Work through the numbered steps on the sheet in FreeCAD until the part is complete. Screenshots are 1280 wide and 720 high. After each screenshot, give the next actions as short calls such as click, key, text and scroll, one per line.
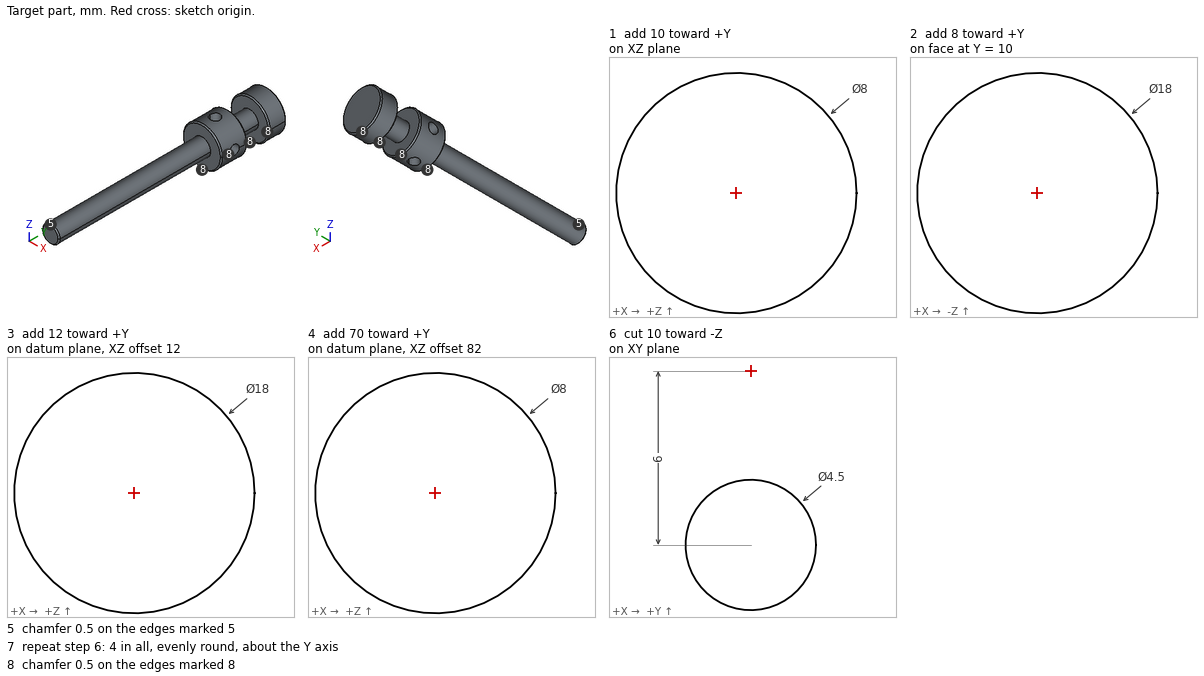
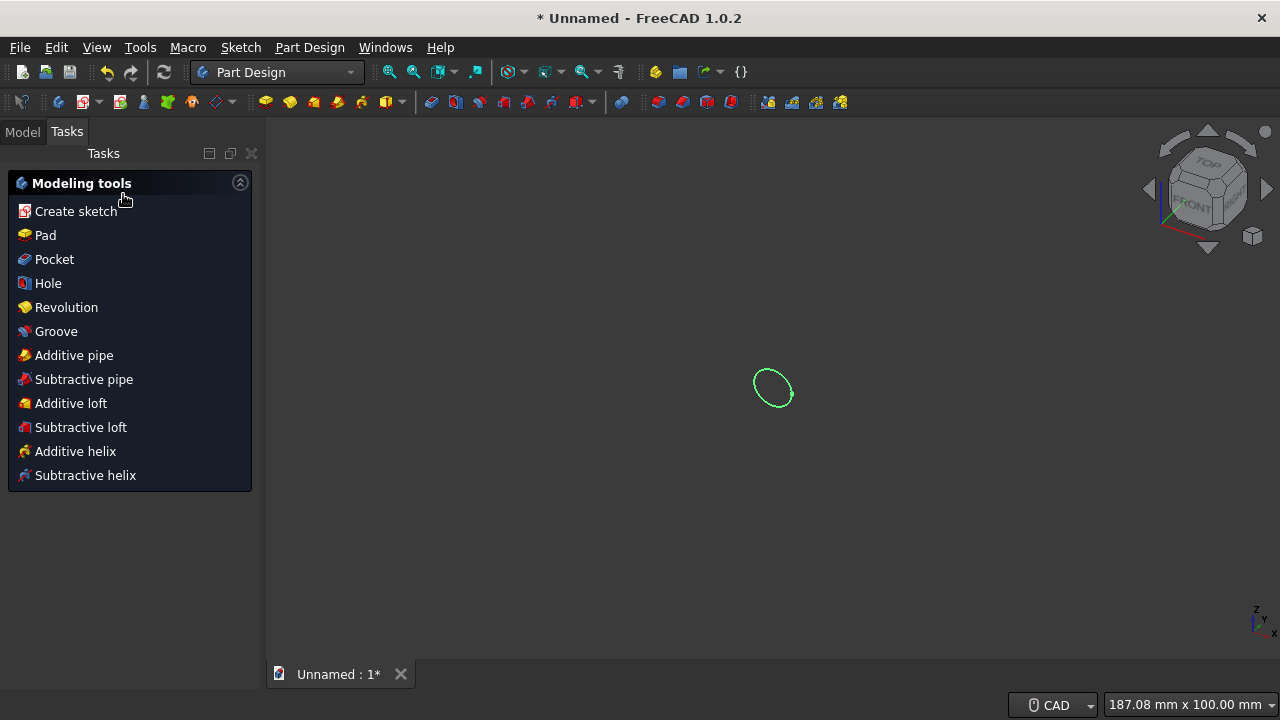
click(266, 102)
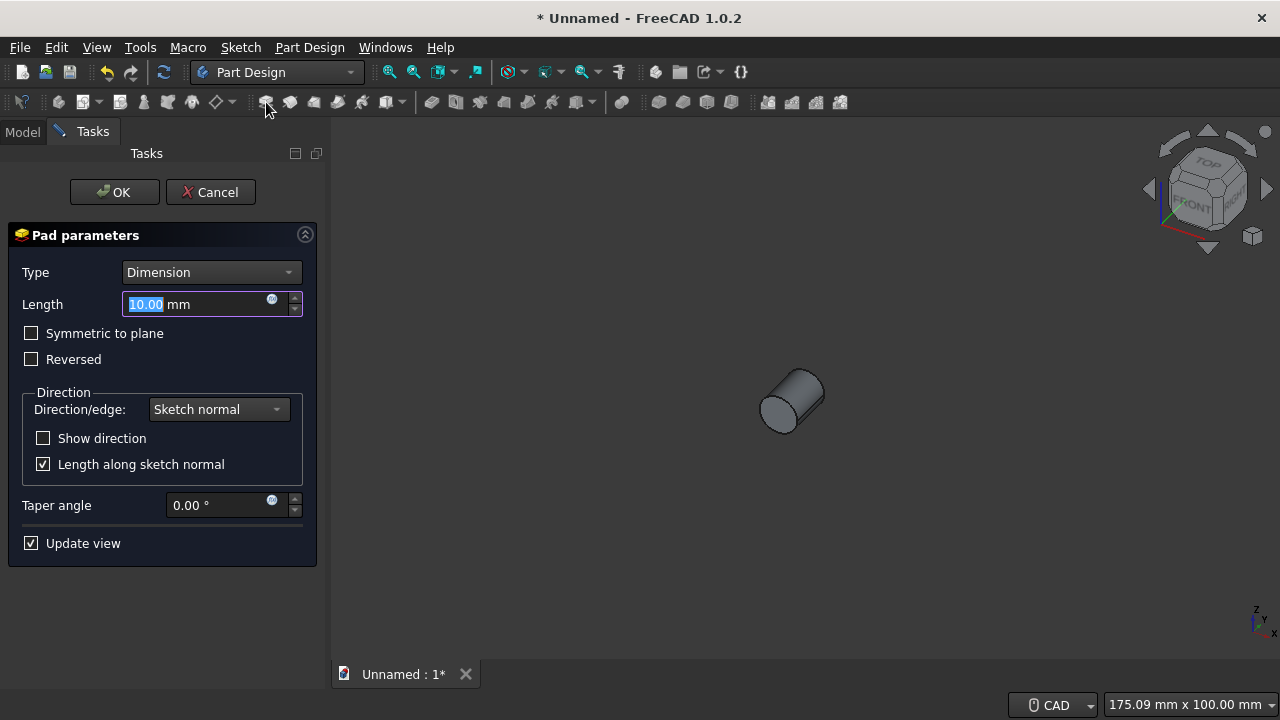
text(10)
key(Tab)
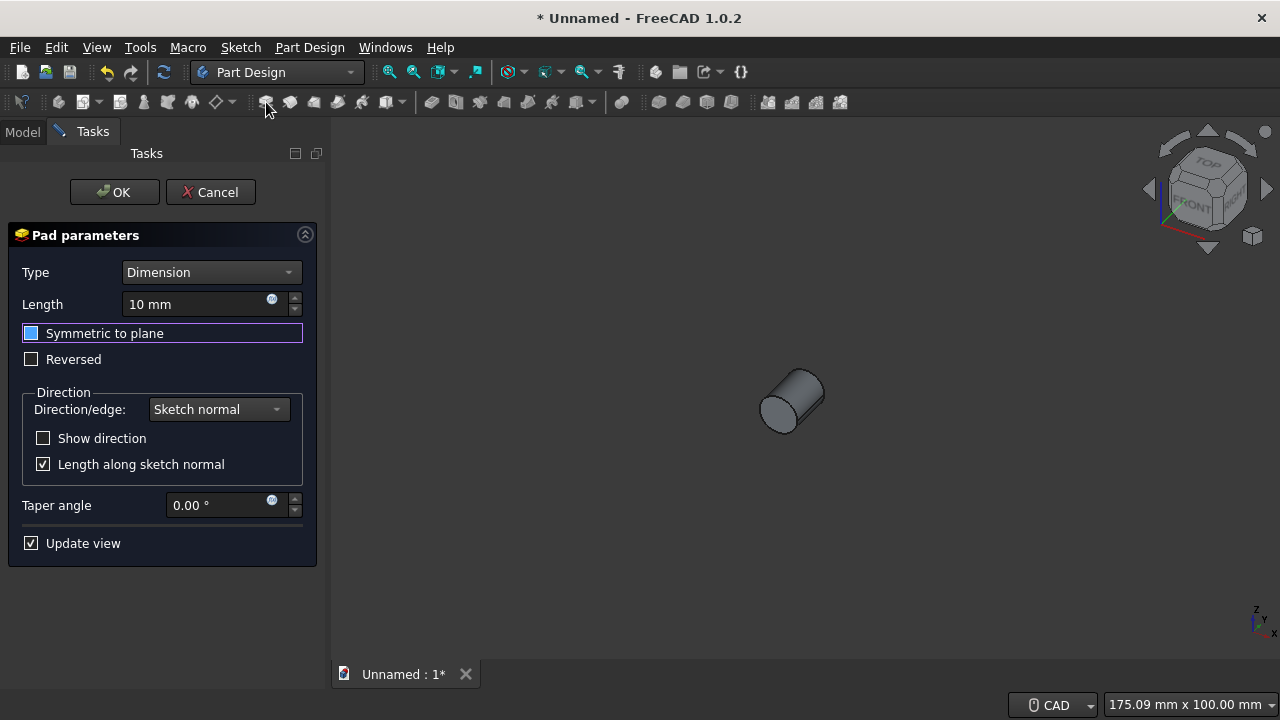
click(30, 359)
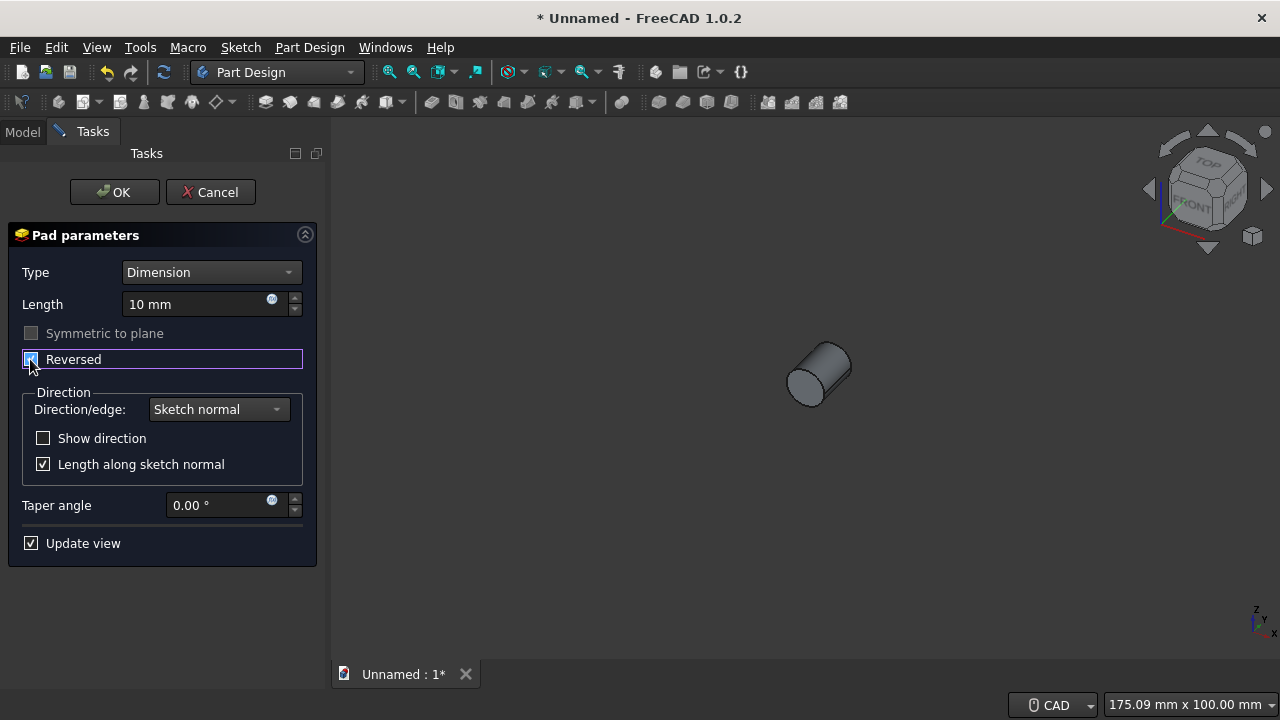
click(115, 192)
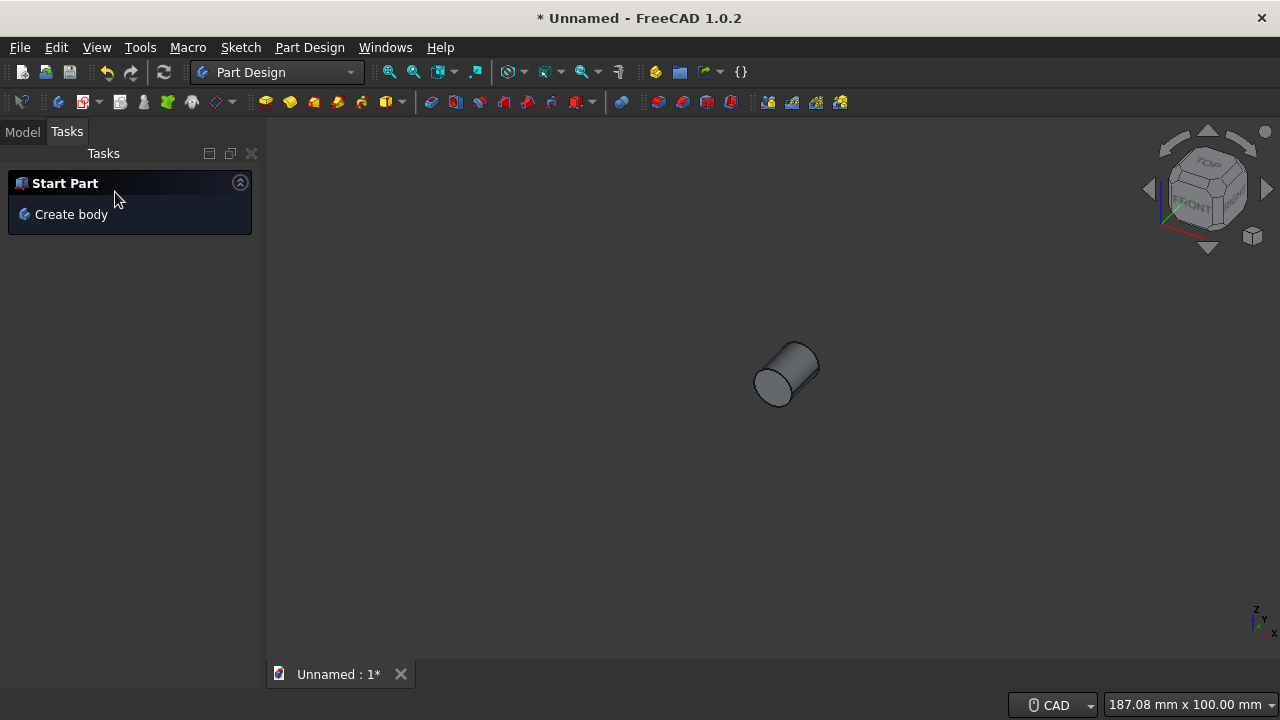
click(390, 72)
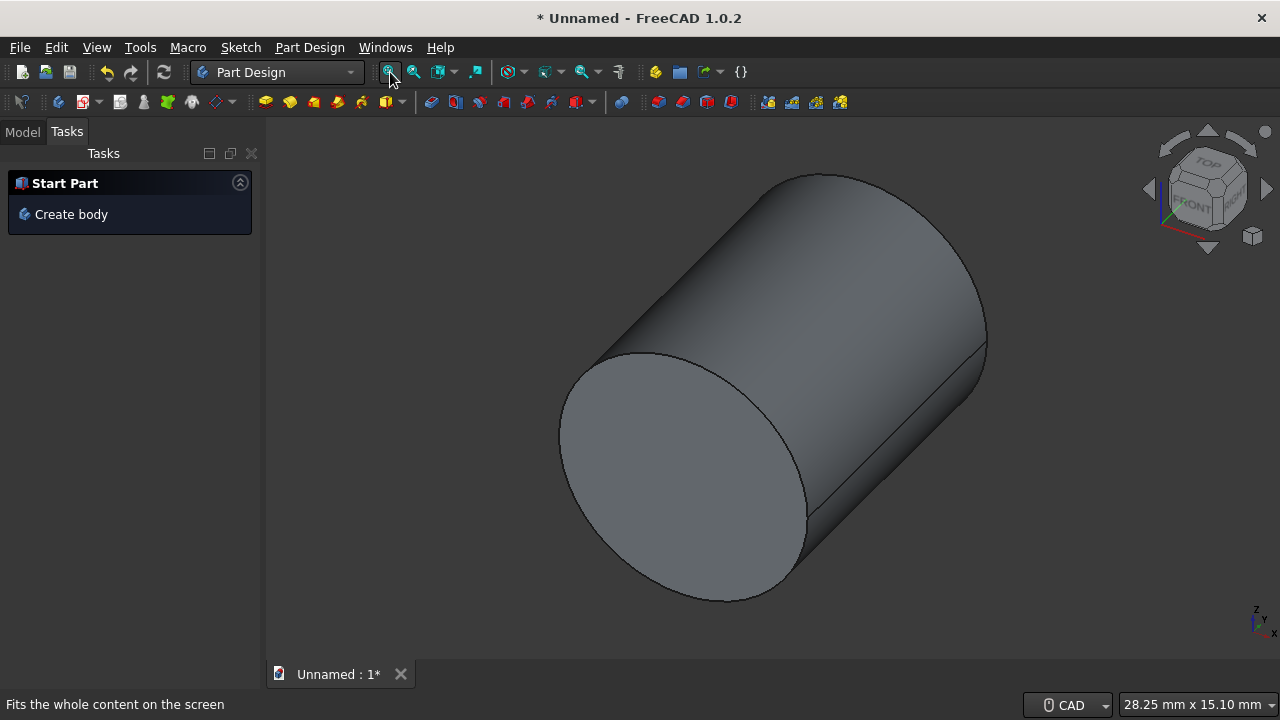
key(4)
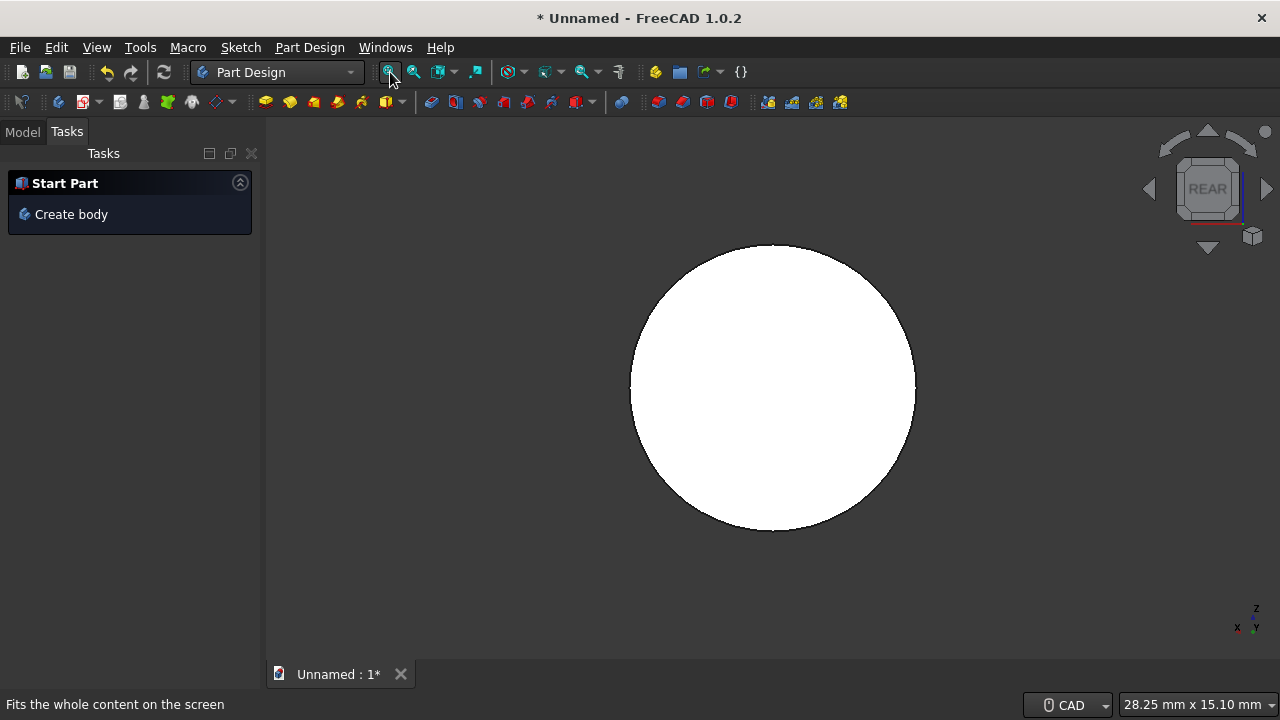
click(773, 387)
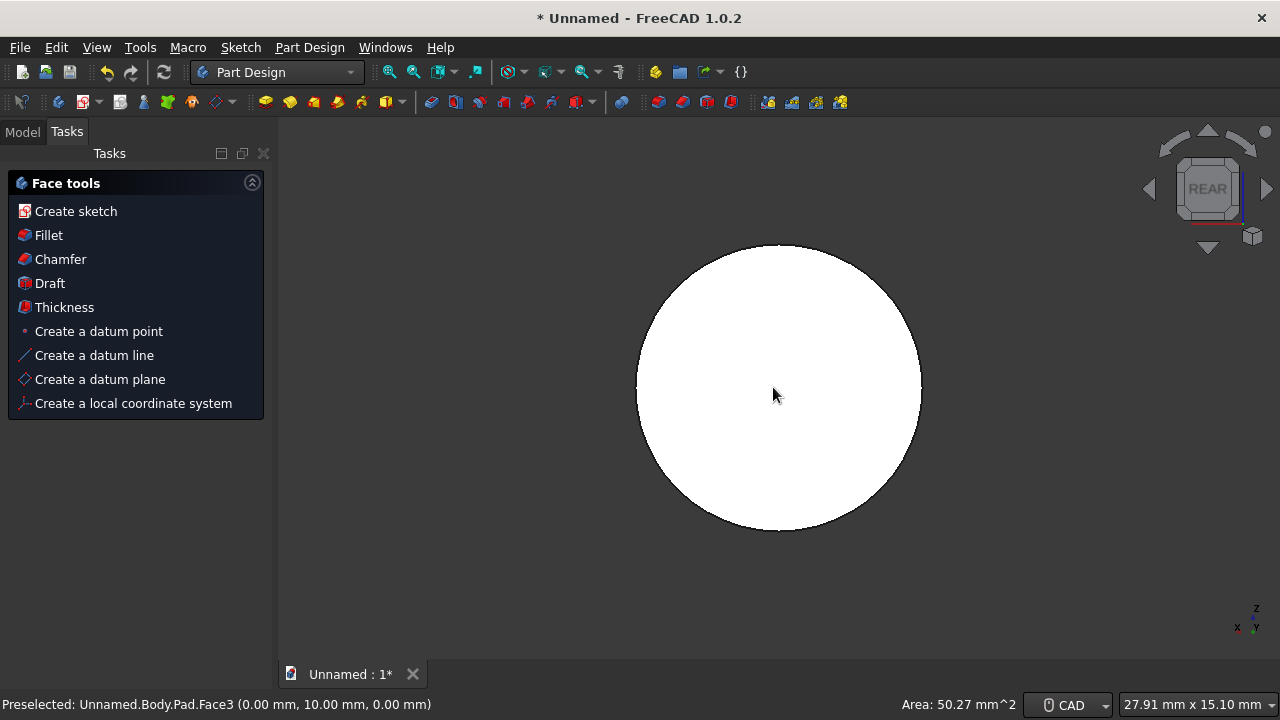
click(84, 102)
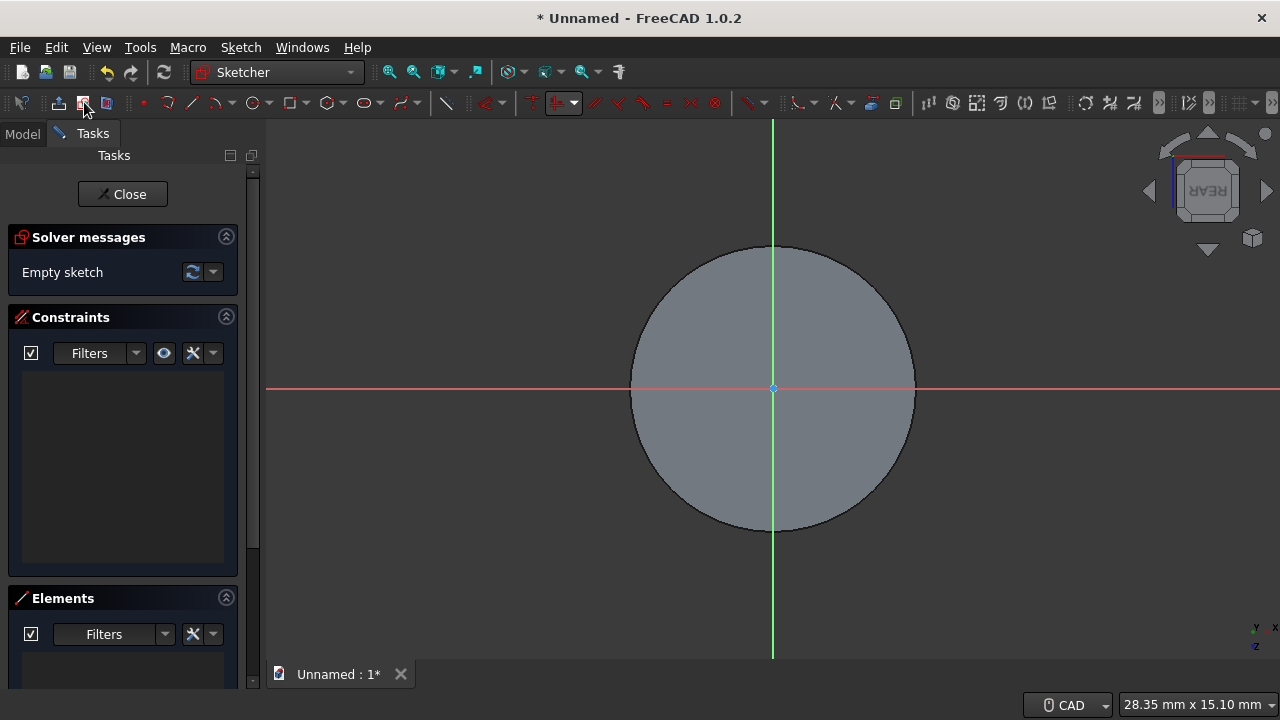
scroll(621, 389, down, 3)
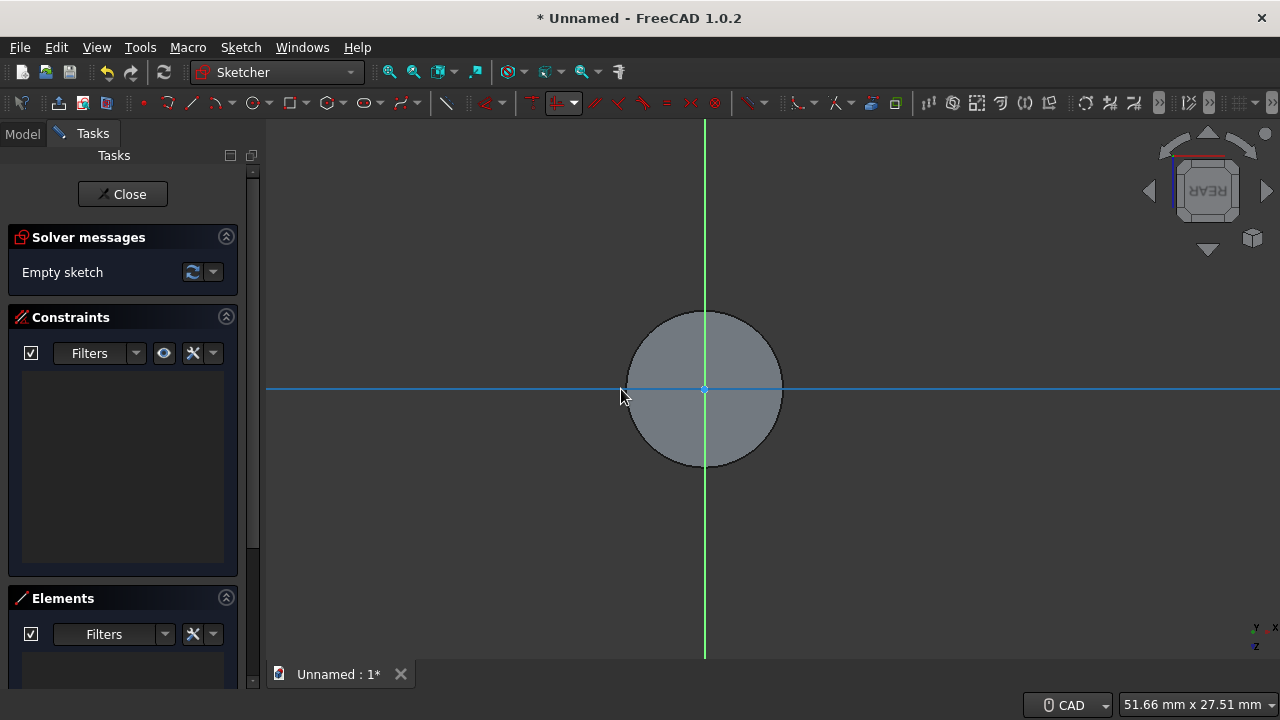
click(254, 104)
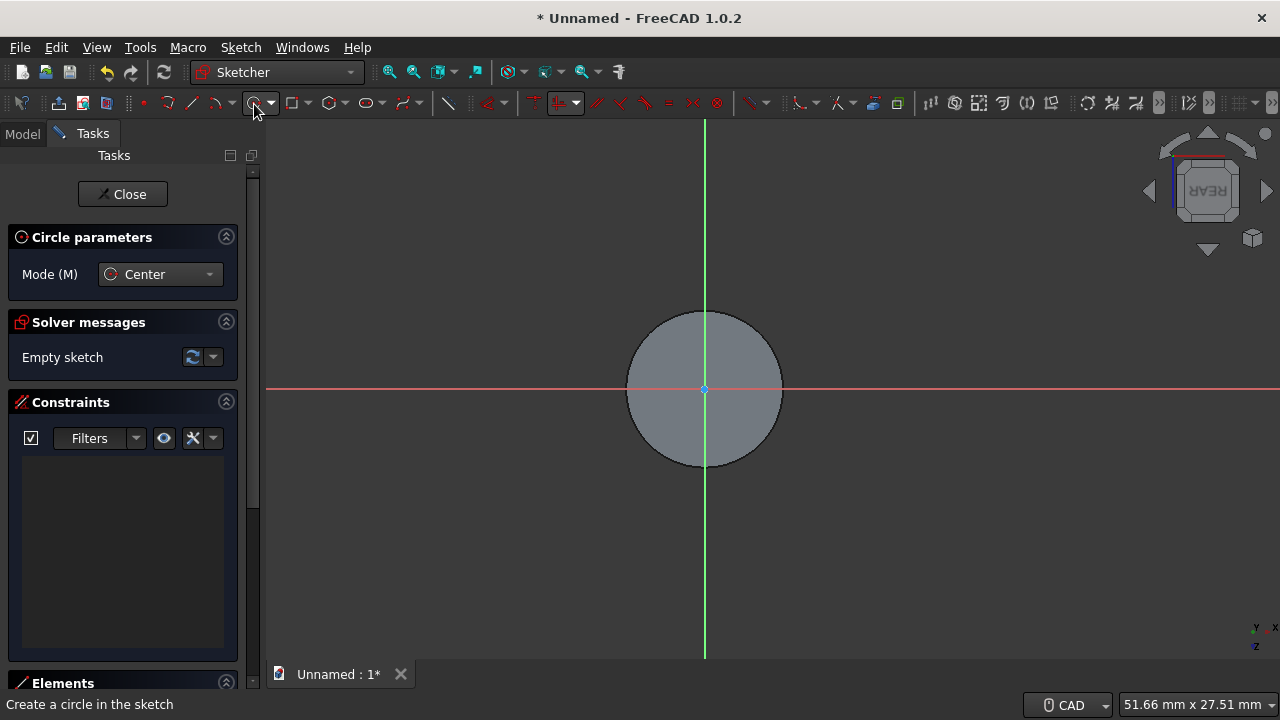
click(705, 389)
click(829, 264)
key(Escape)